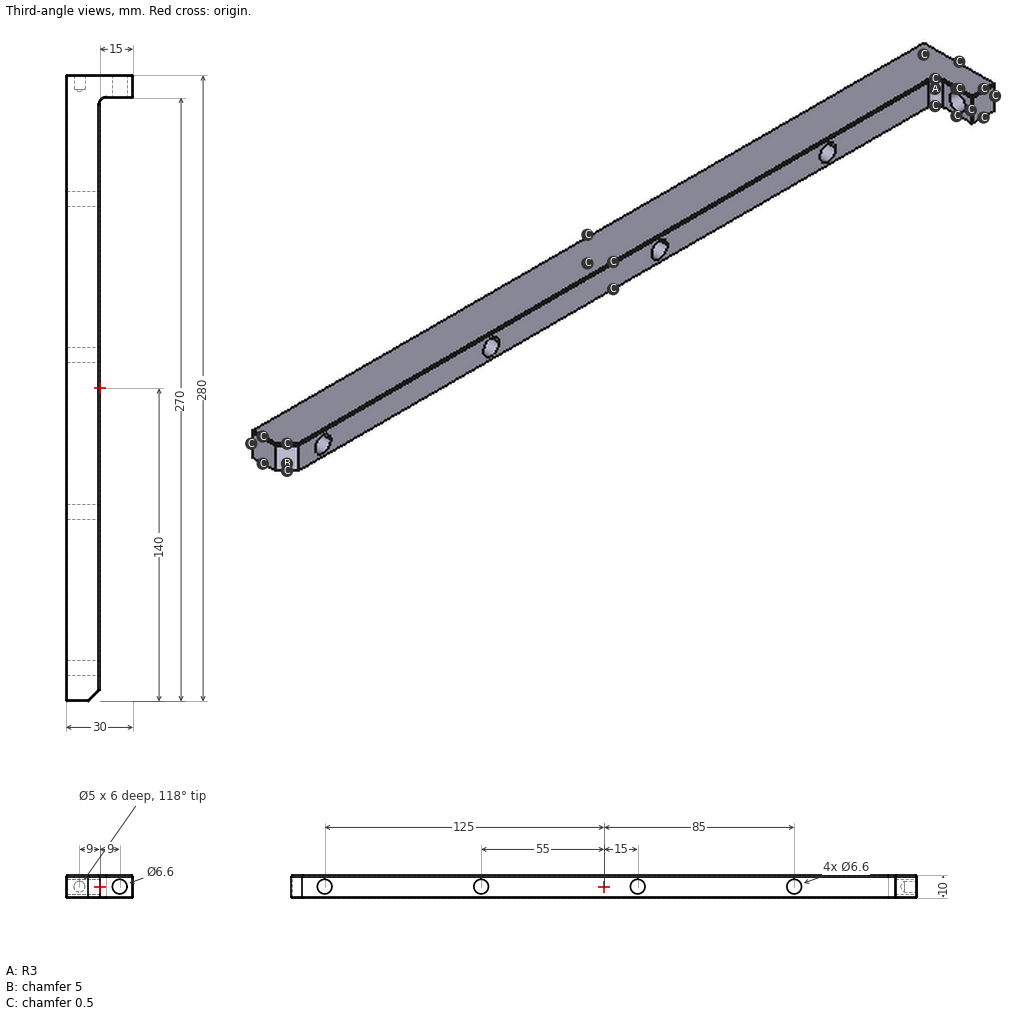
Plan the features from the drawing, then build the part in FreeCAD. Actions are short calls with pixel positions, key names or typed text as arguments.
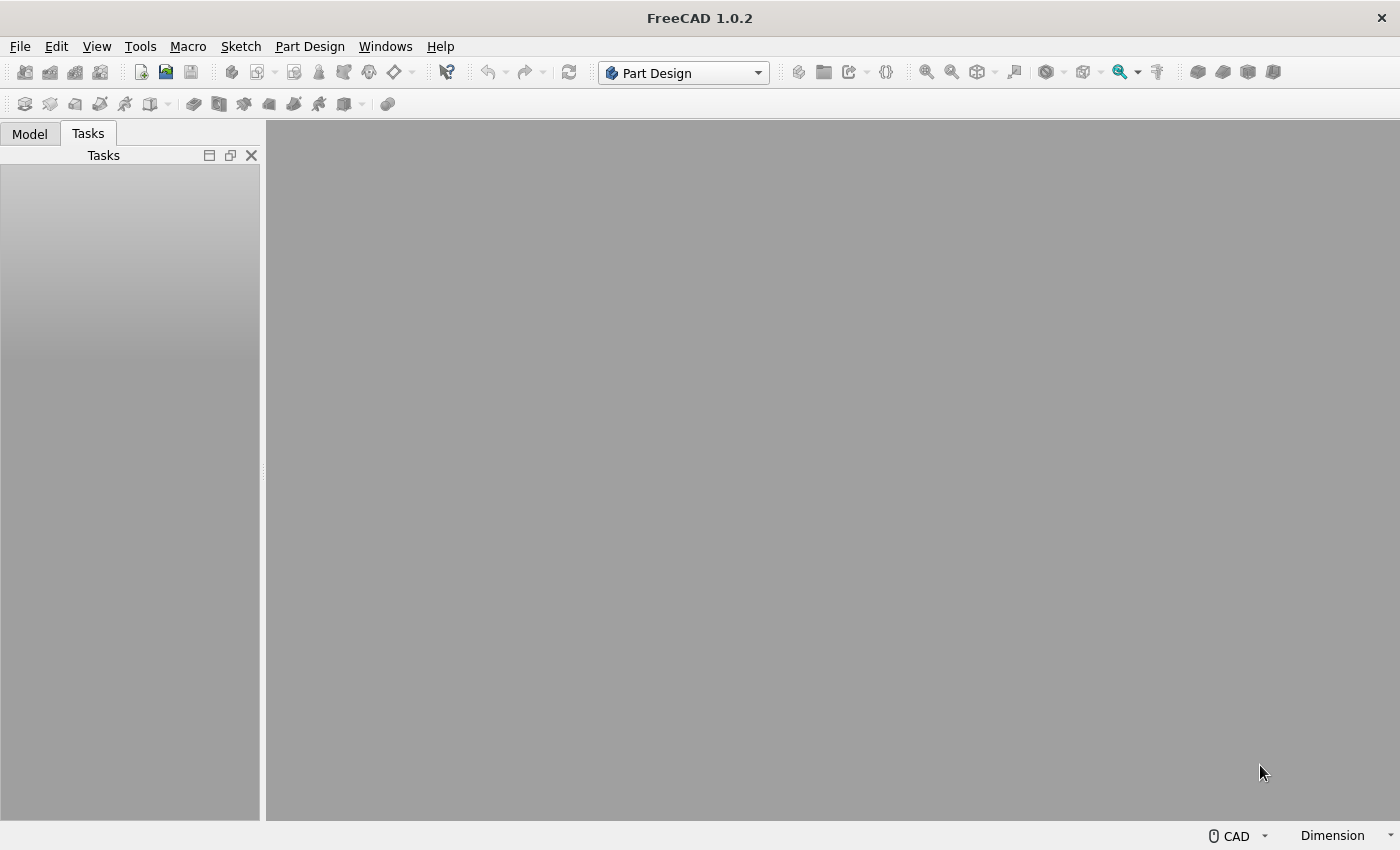
key(ctrl+n)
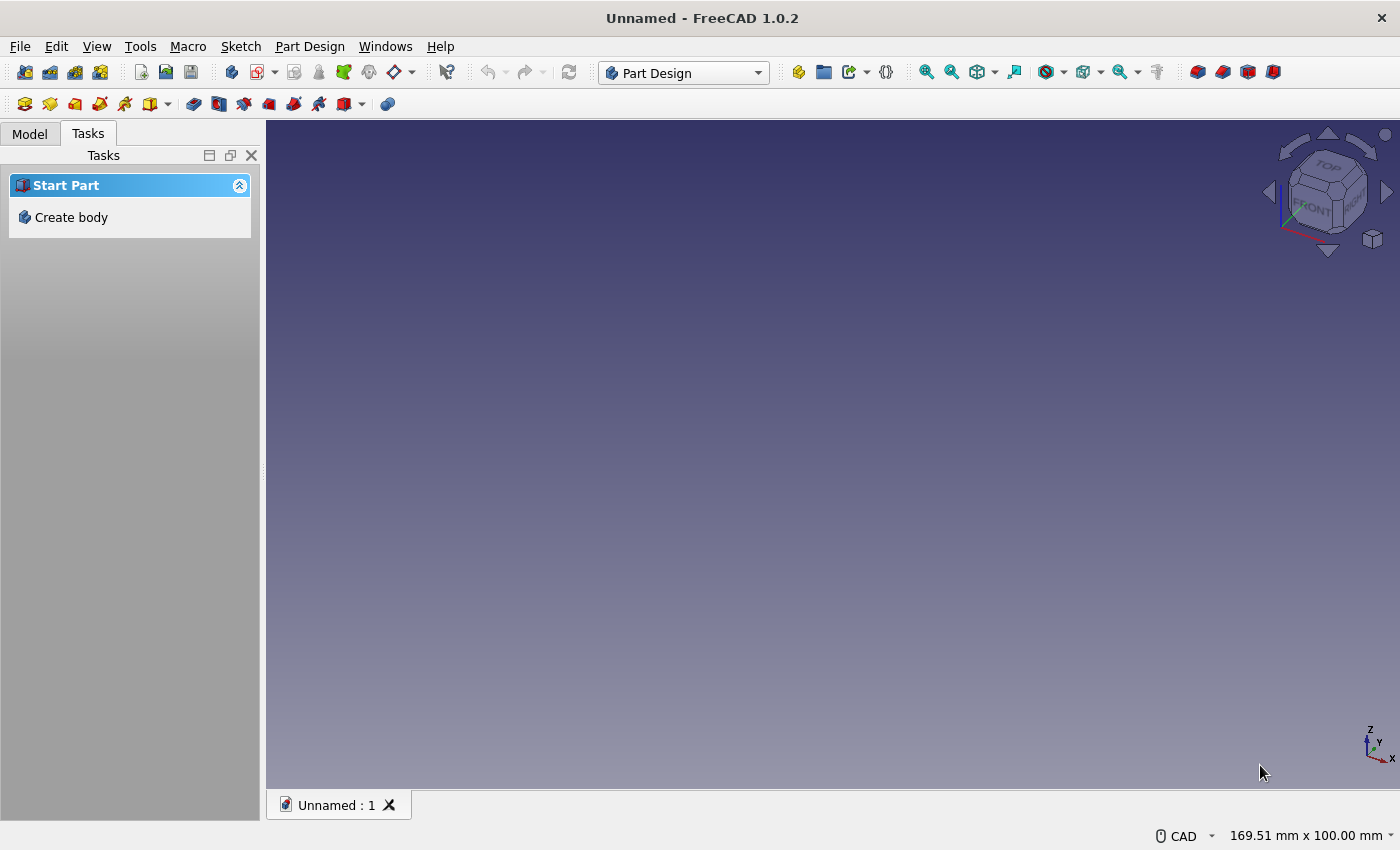
click(256, 72)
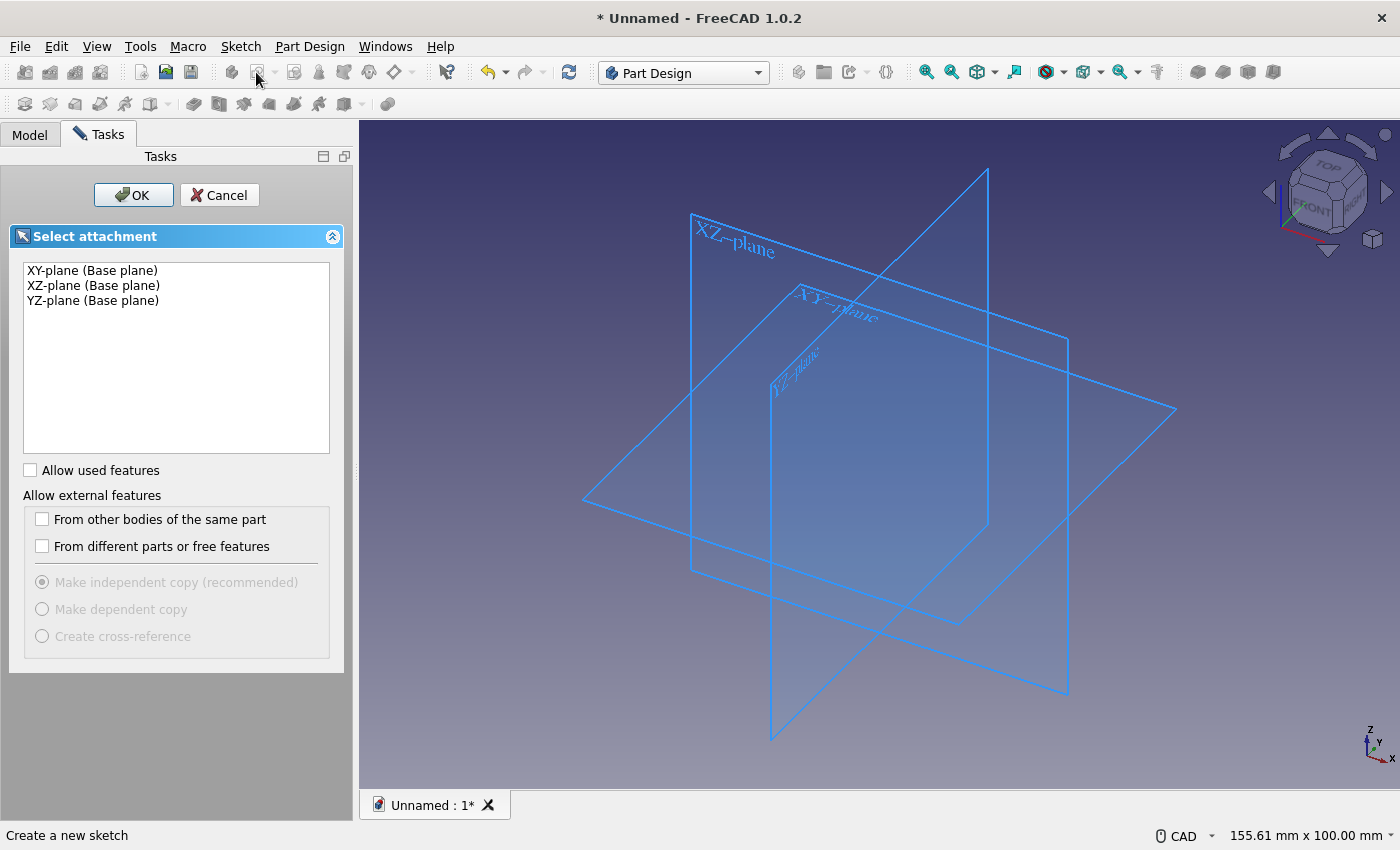
click(84, 270)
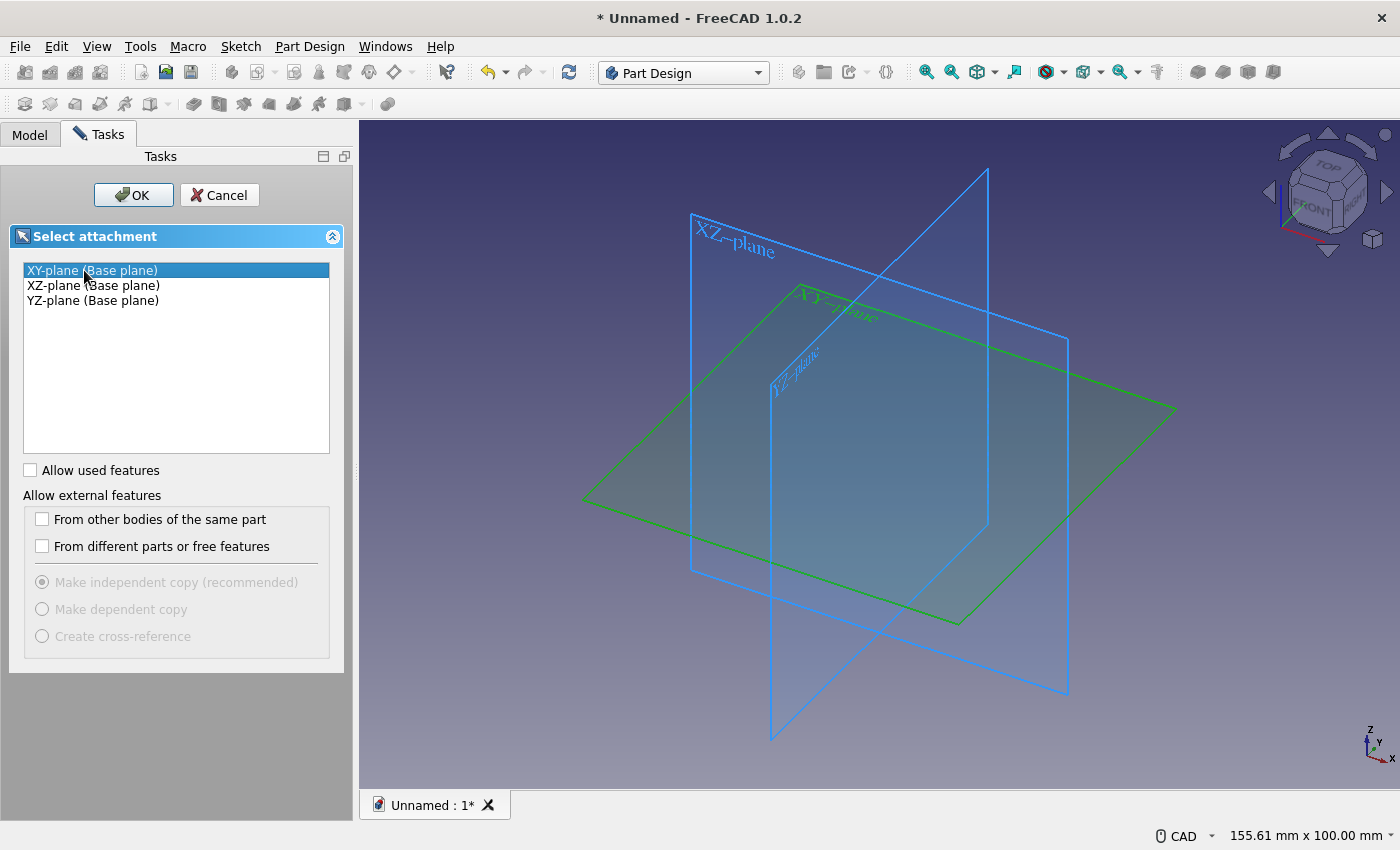
click(134, 195)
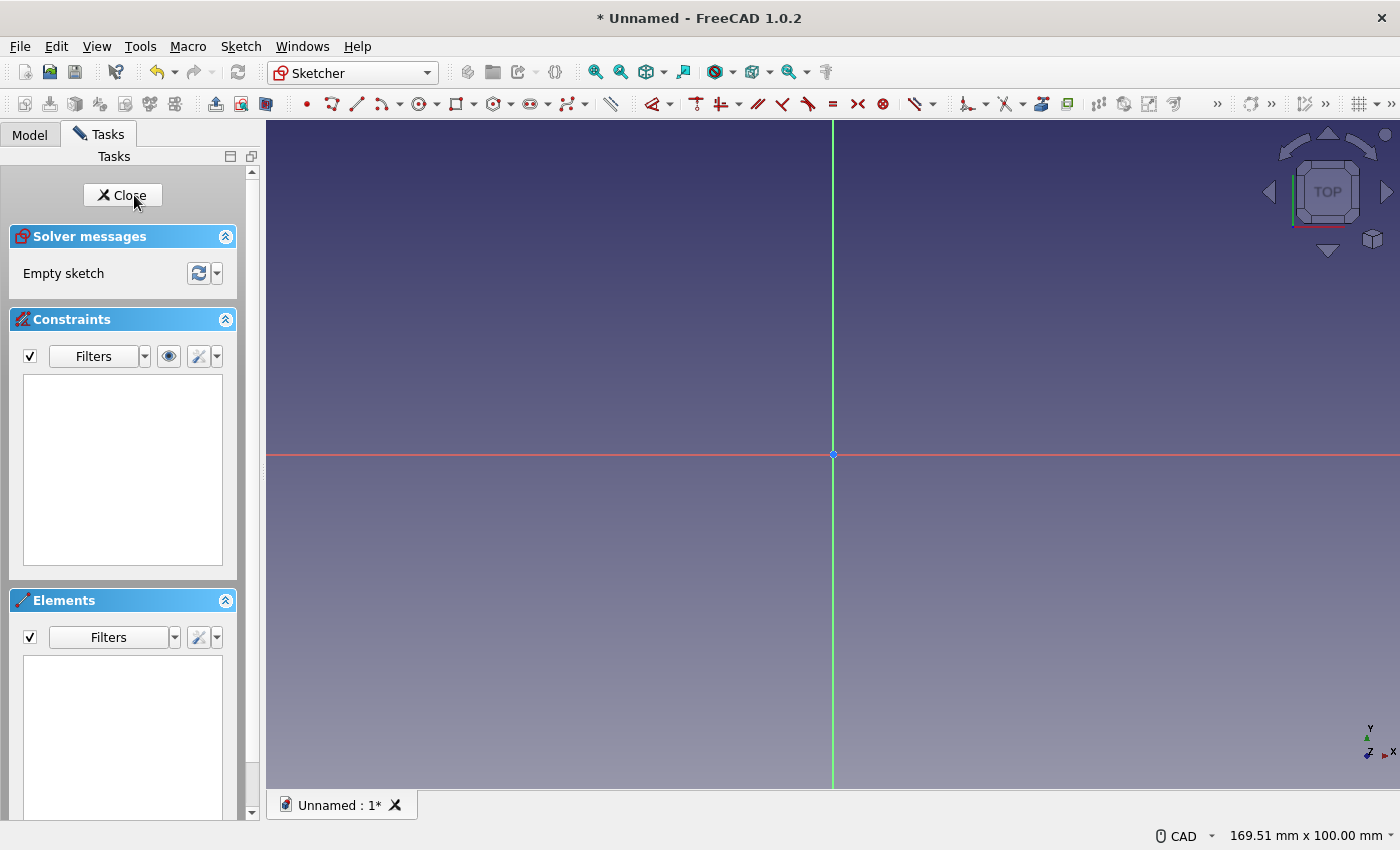
scroll(742, 454, down, 7)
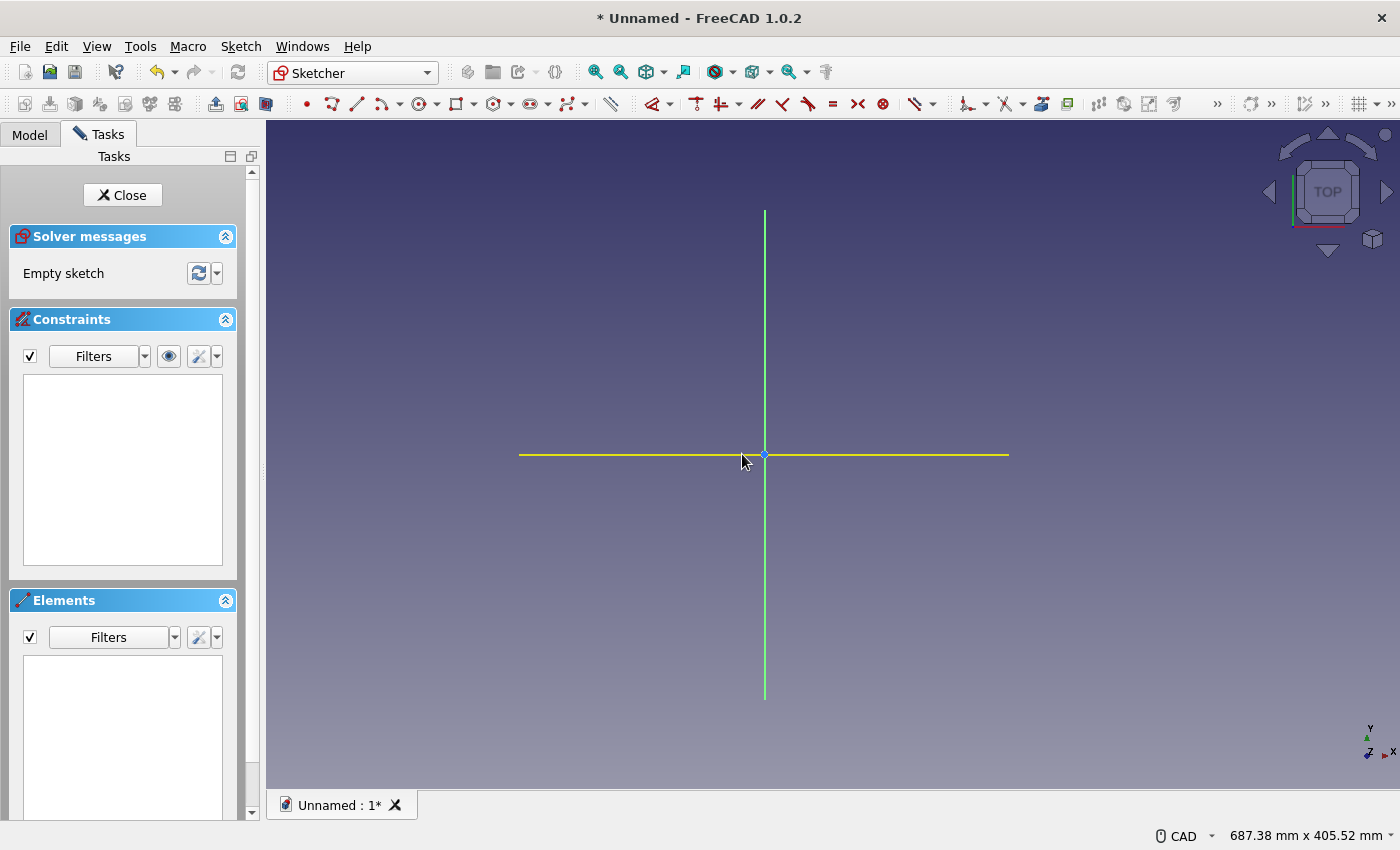
key(g)
key(v)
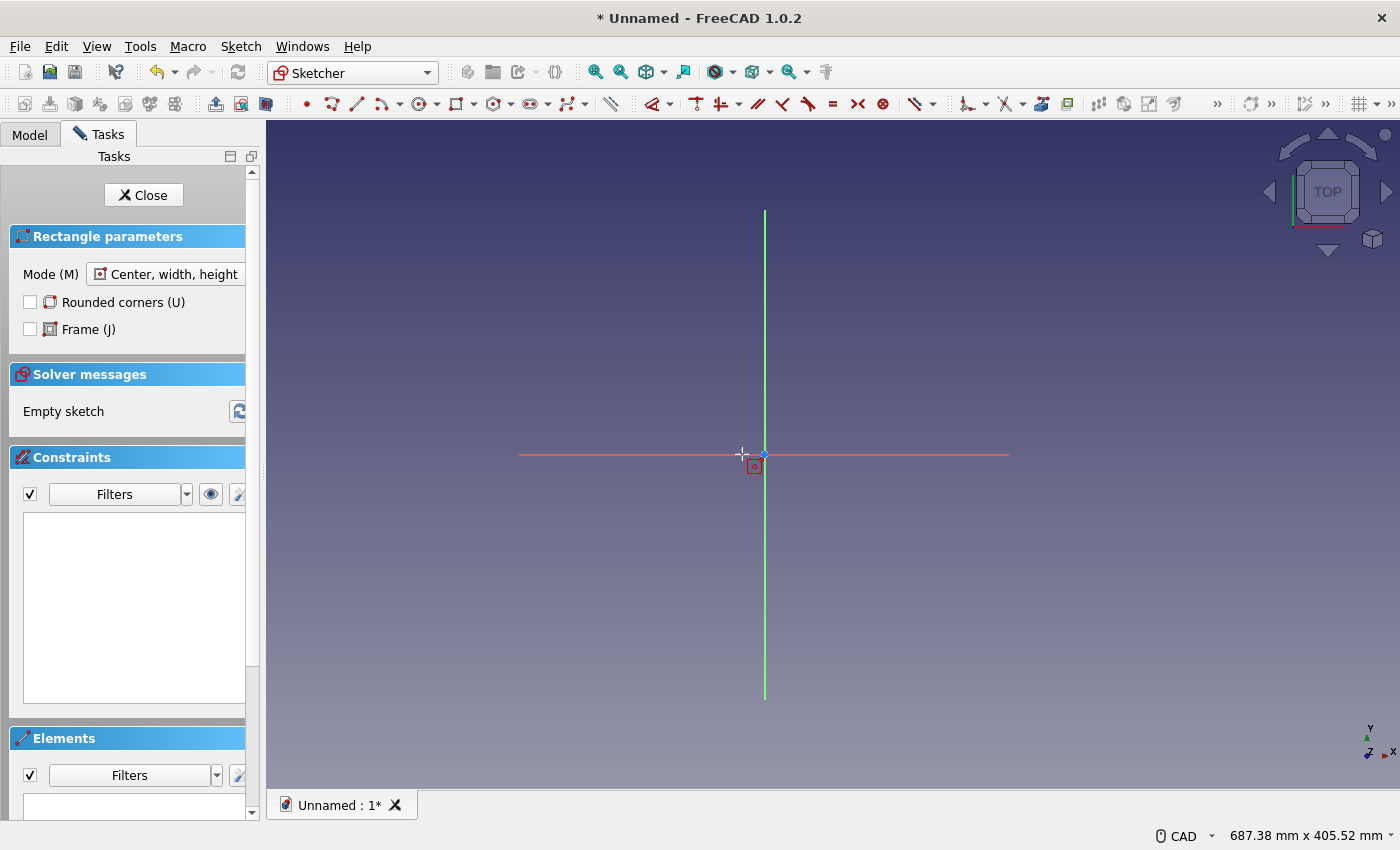
click(765, 454)
click(790, 224)
key(Escape)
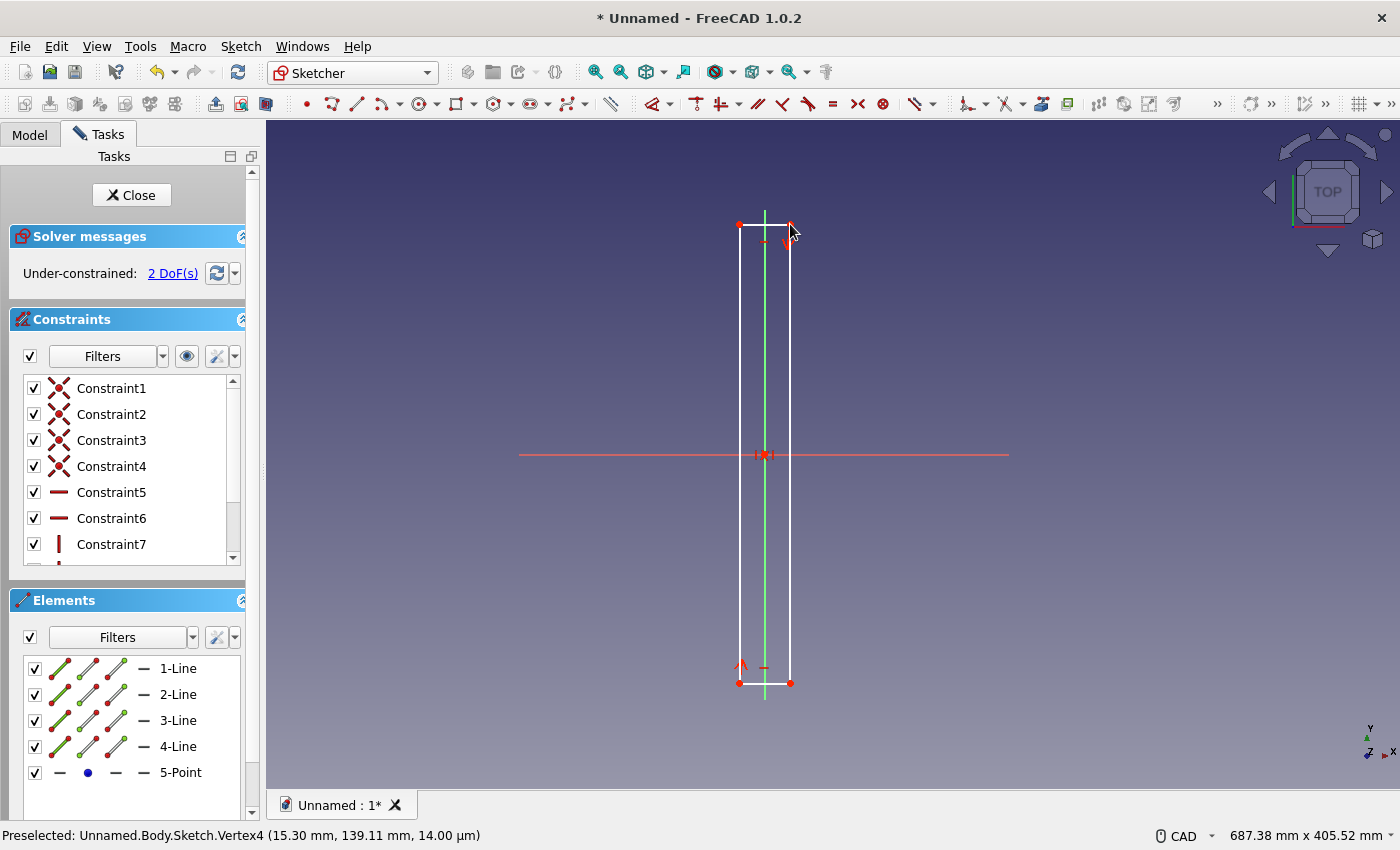
key(d)